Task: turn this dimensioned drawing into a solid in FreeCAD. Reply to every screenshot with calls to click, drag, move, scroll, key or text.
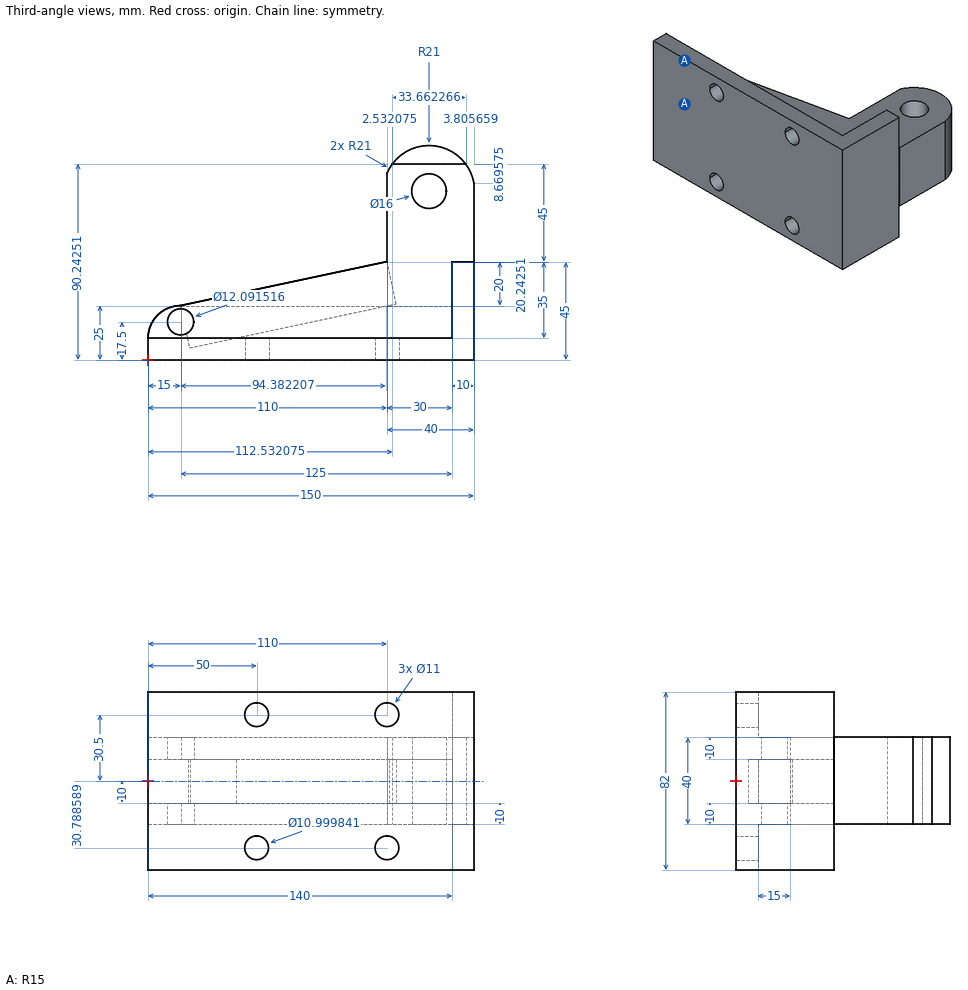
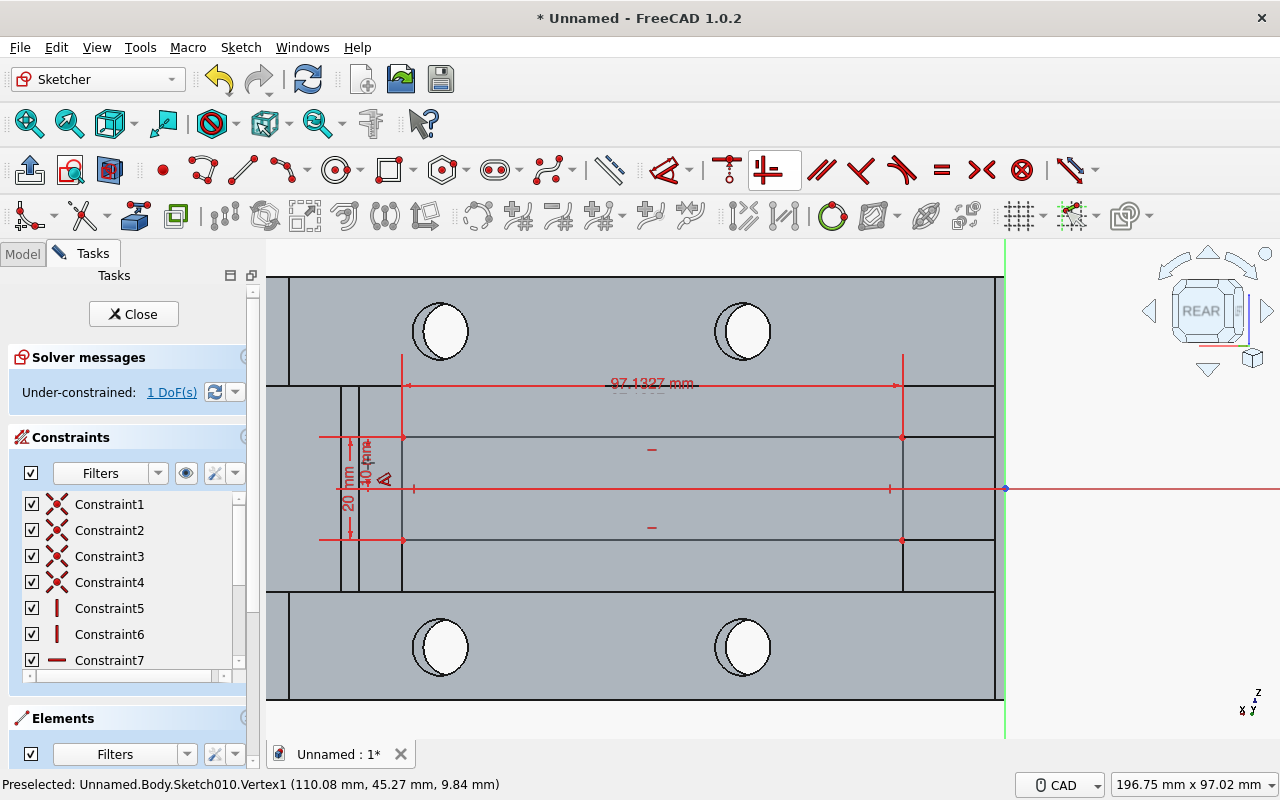
click(903, 540)
click(954, 574)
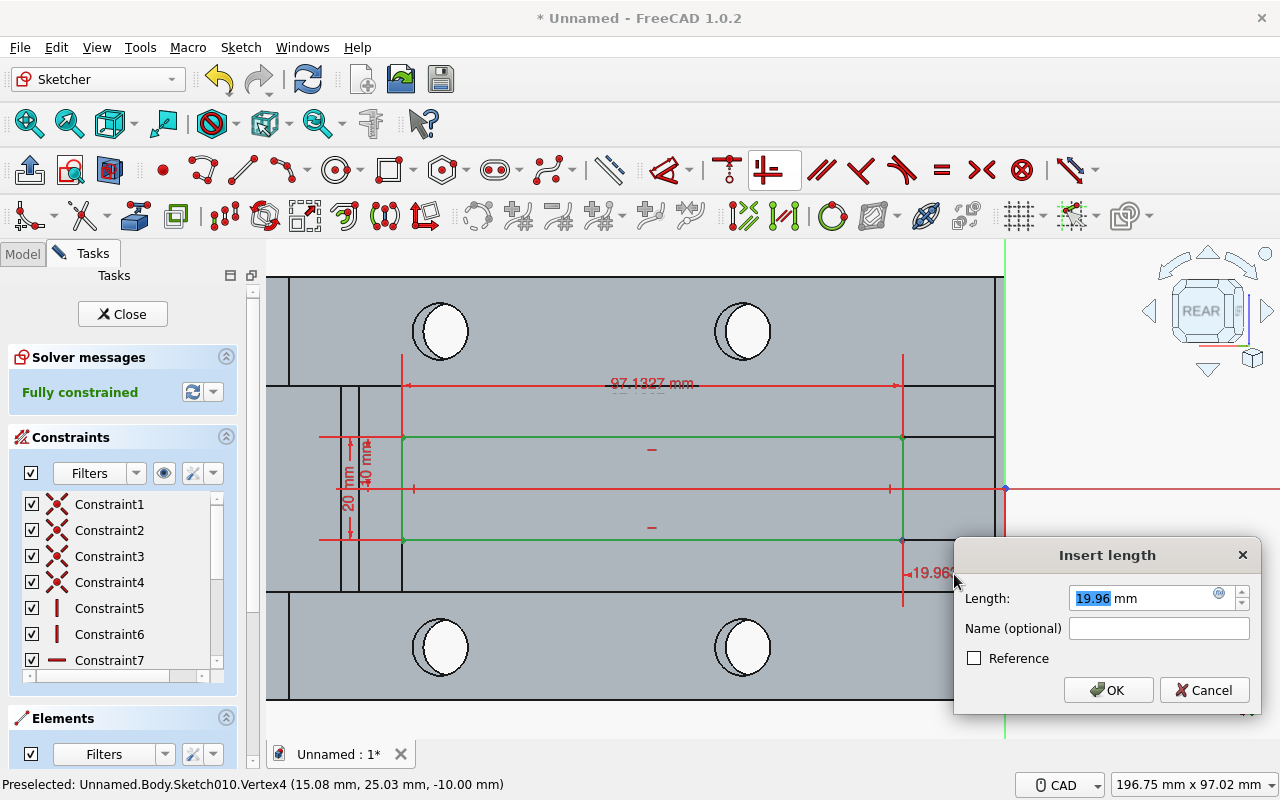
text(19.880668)
key(Return)
key(Escape)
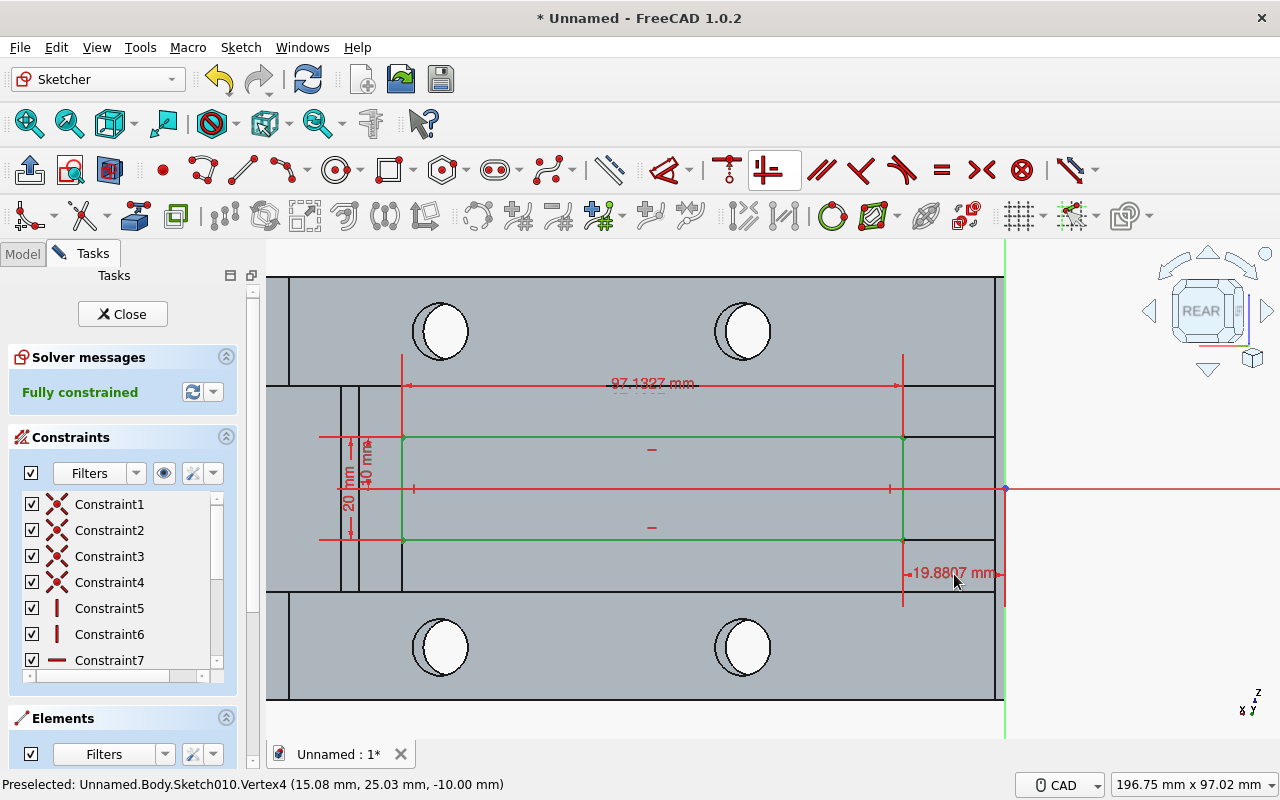
click(123, 314)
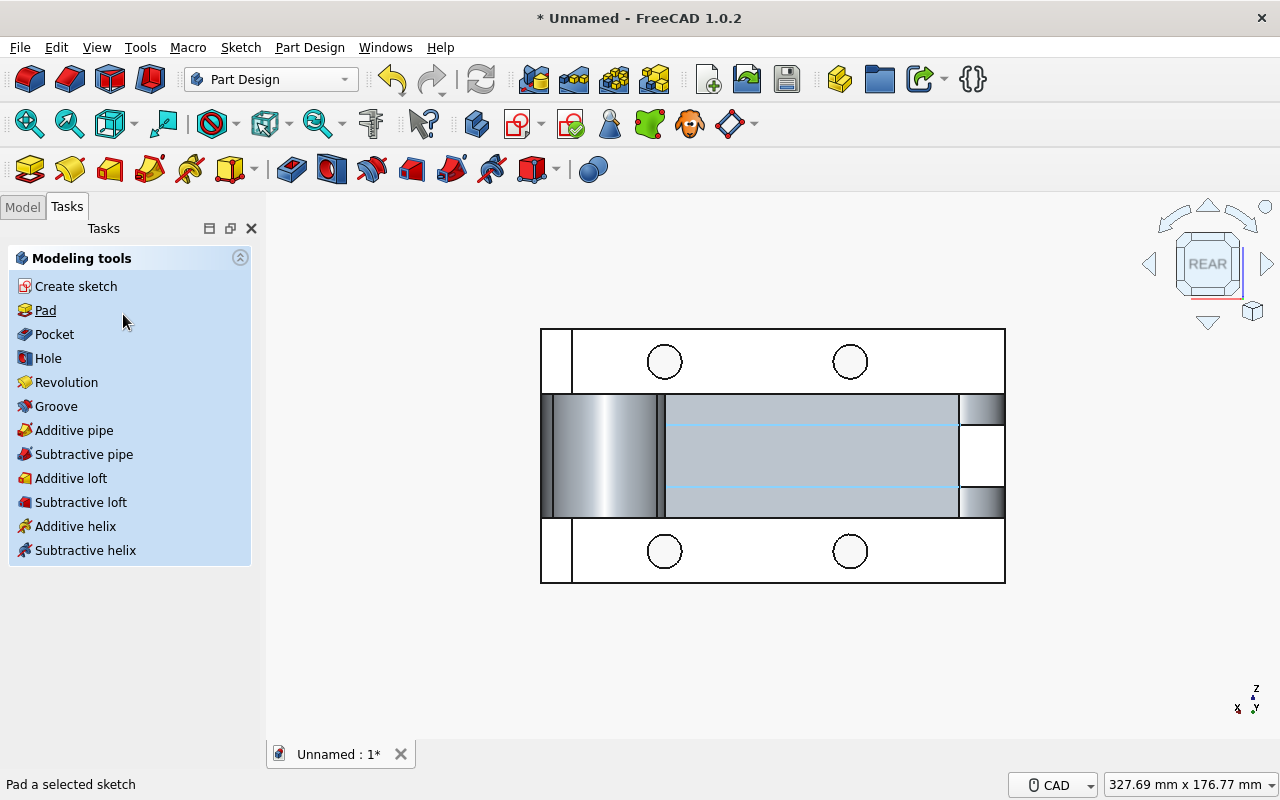
click(292, 170)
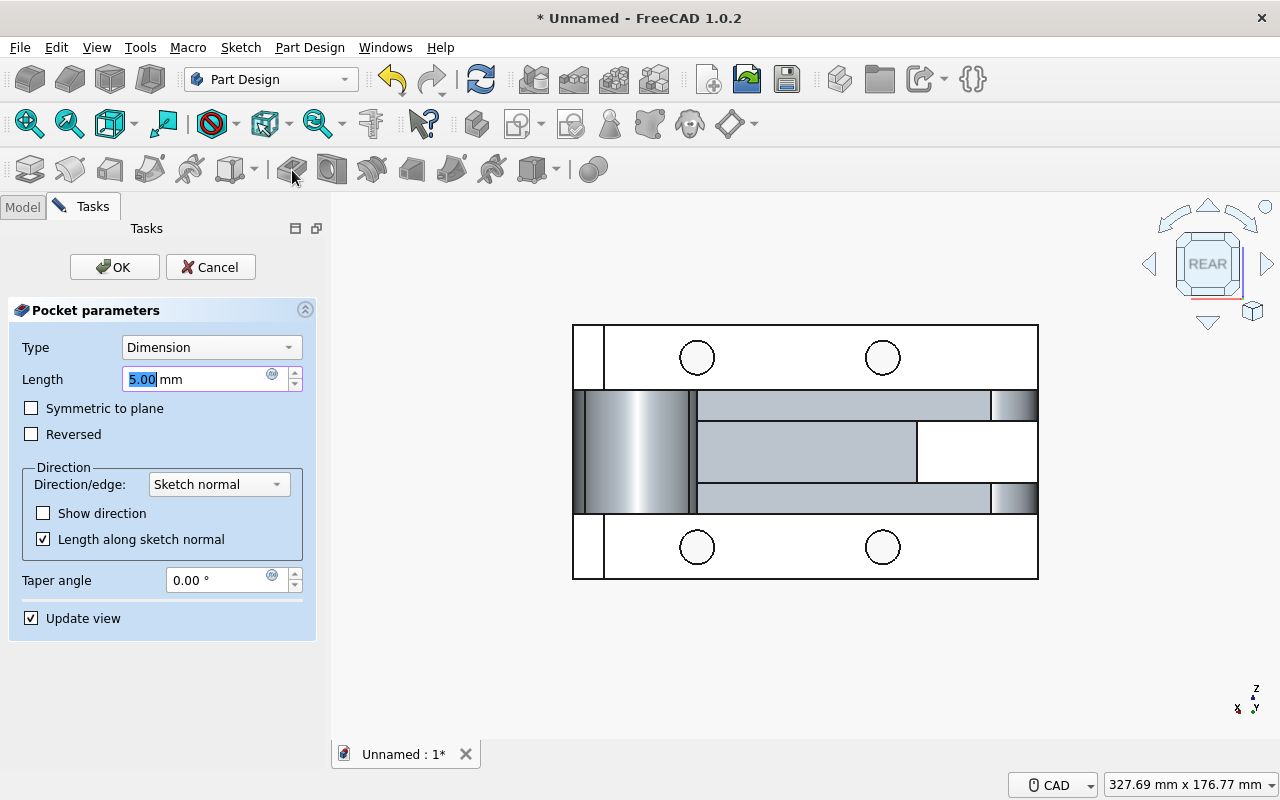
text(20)
key(Tab)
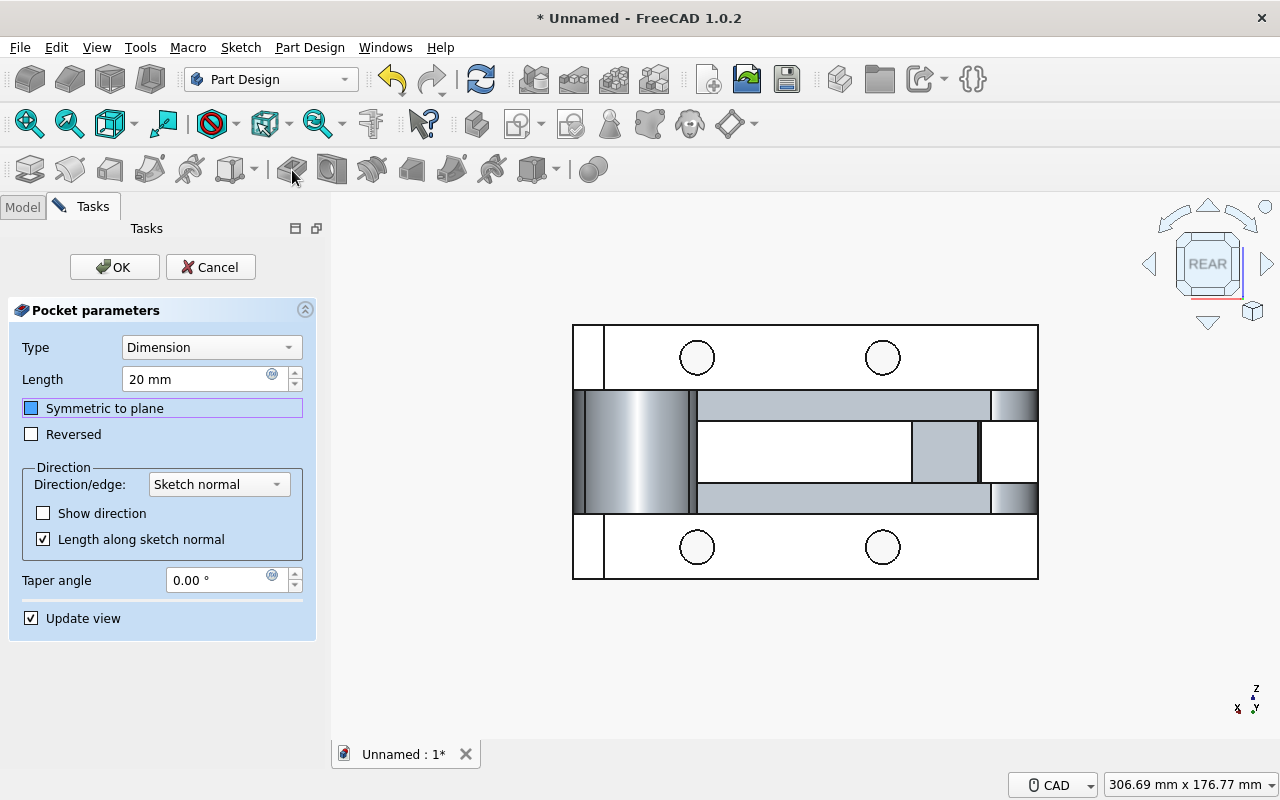
click(115, 267)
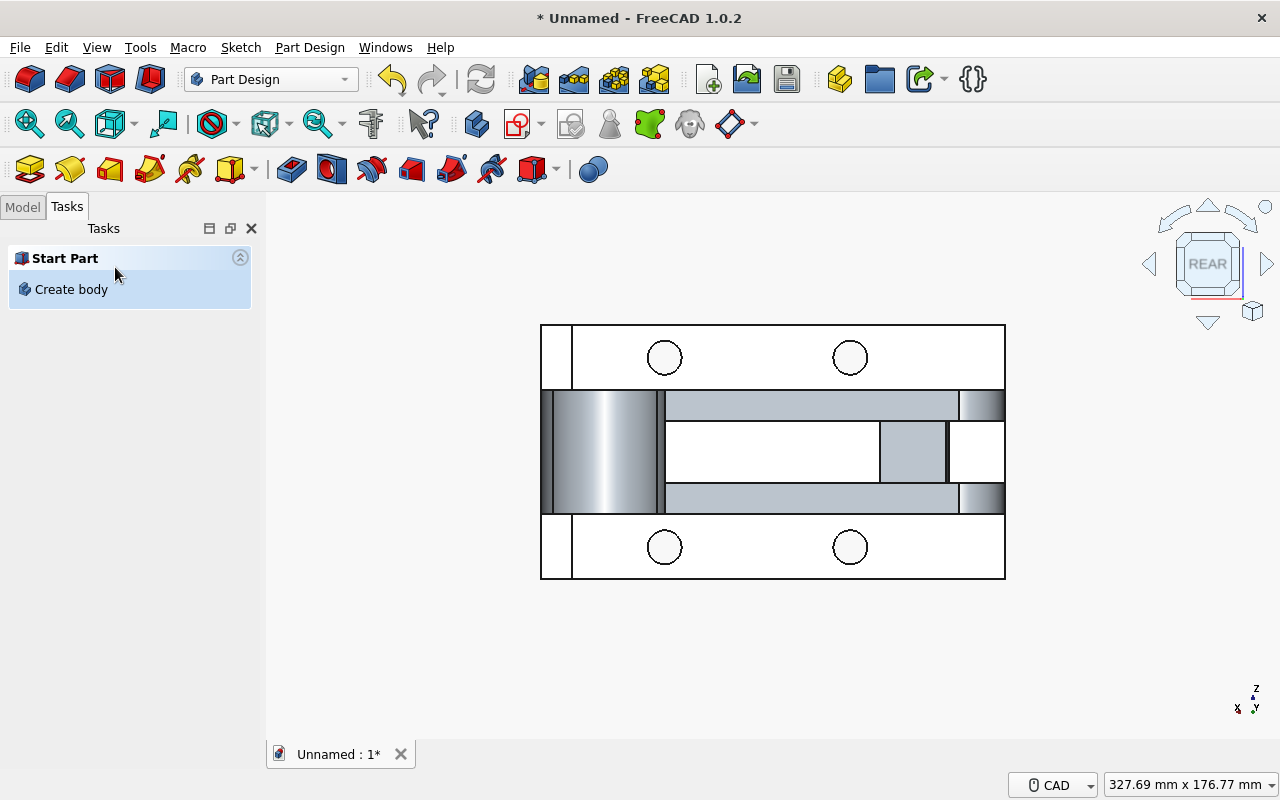
key(0)